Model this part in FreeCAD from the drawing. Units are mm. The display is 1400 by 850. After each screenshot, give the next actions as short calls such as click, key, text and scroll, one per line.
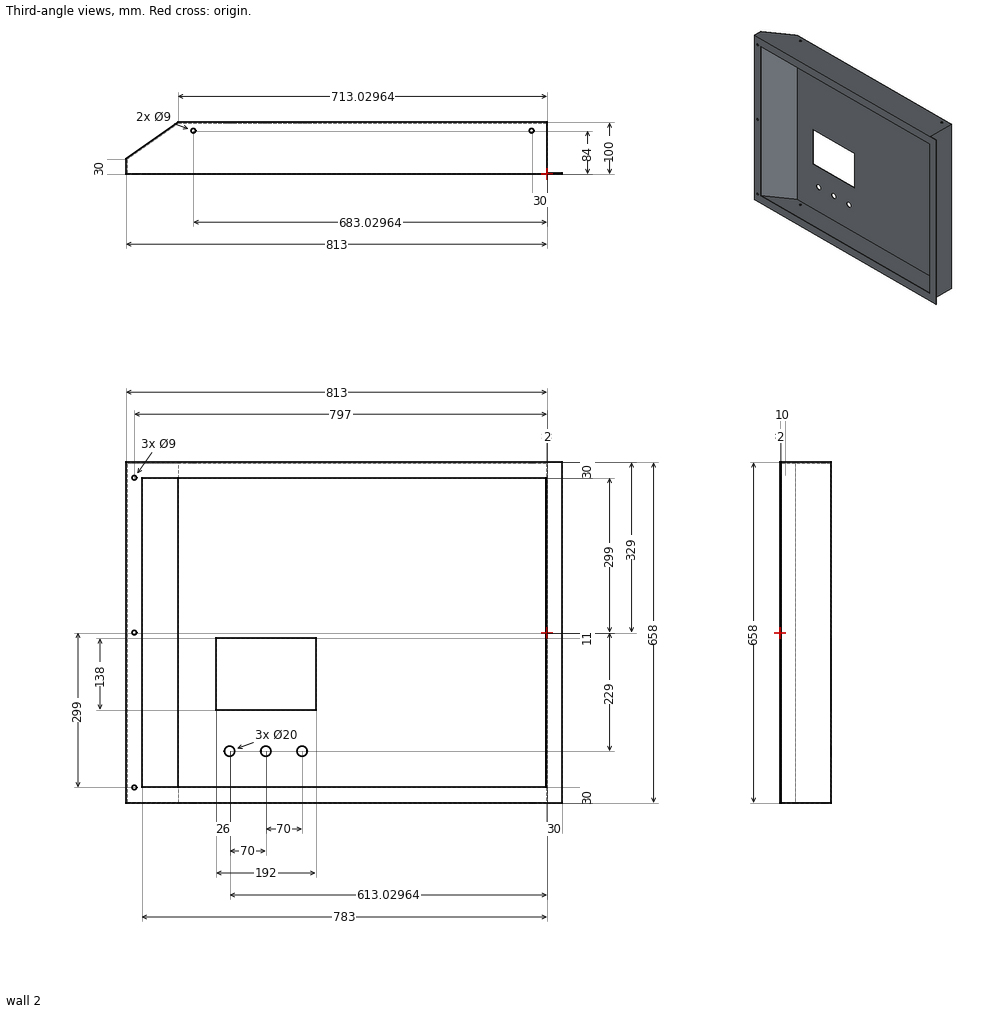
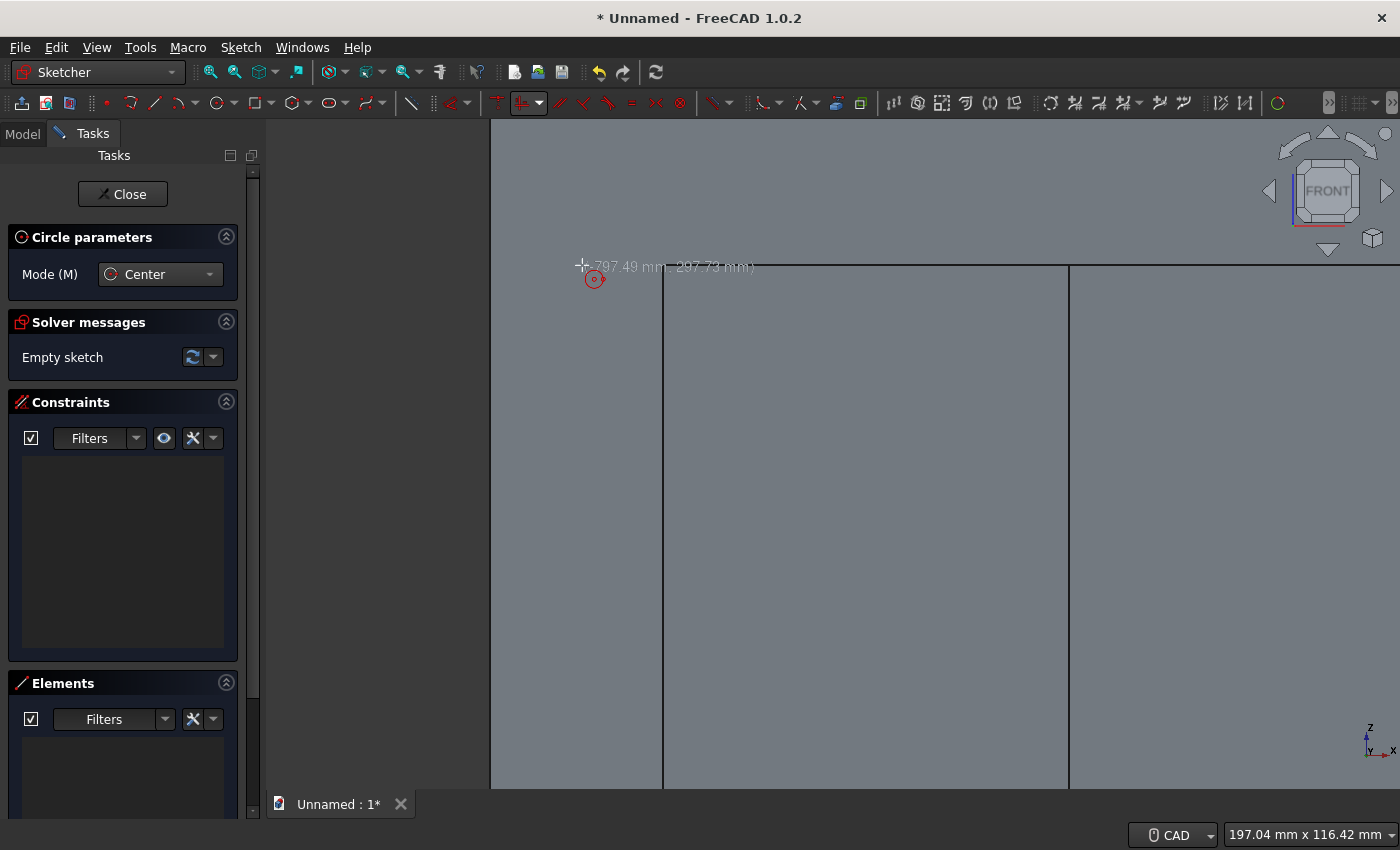
scroll(436, 214, down, 10)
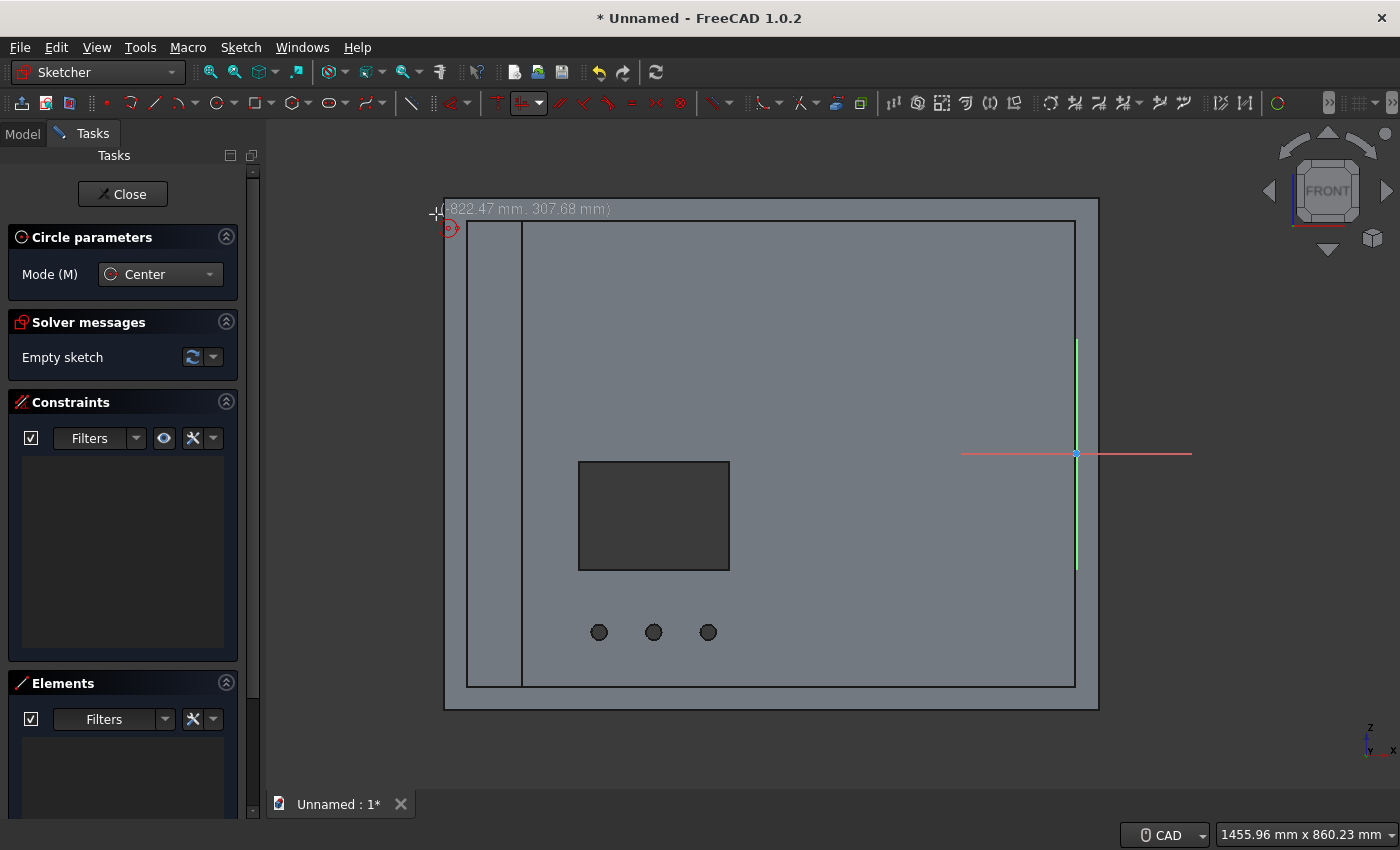
click(456, 221)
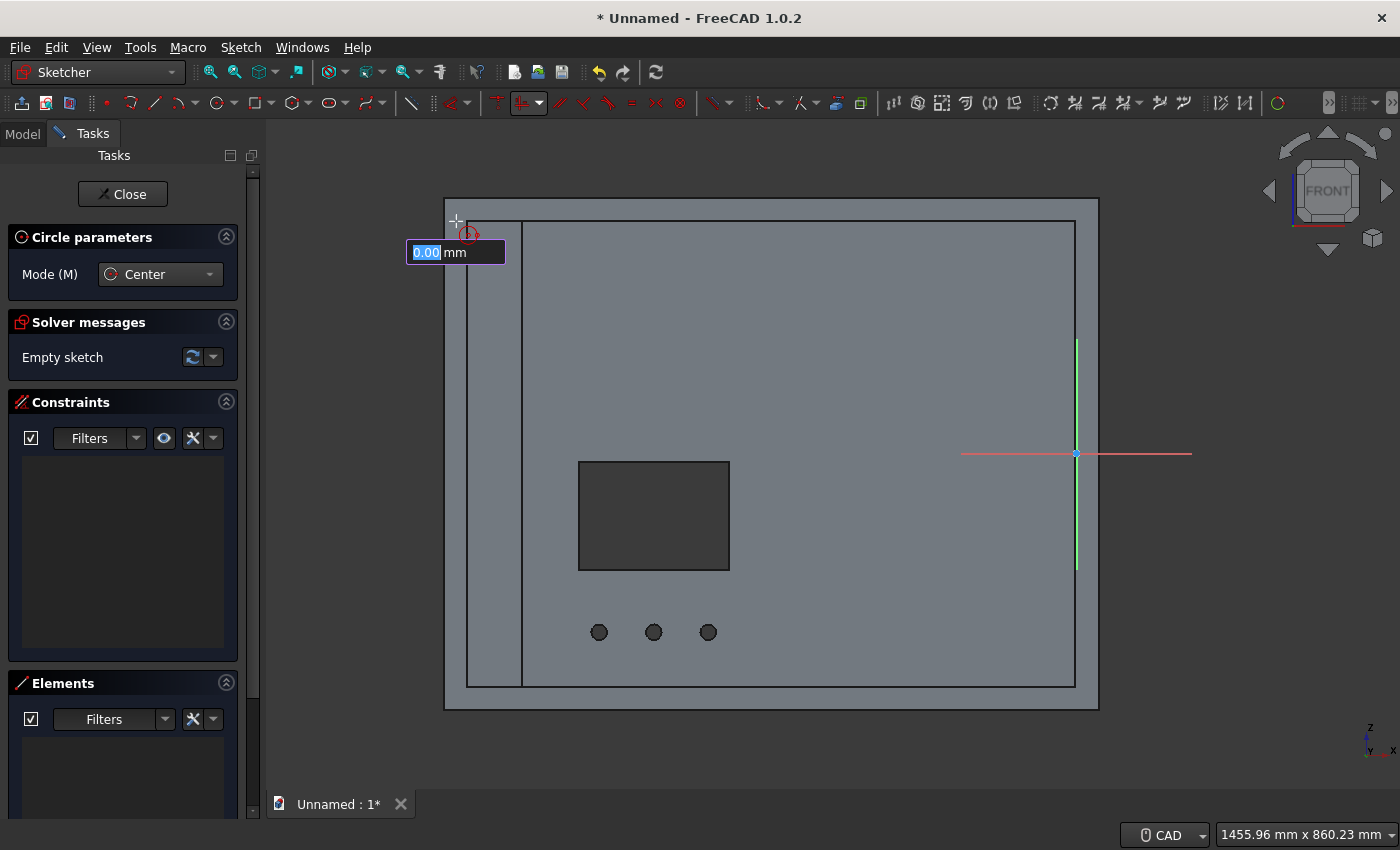
scroll(458, 219, up, 8)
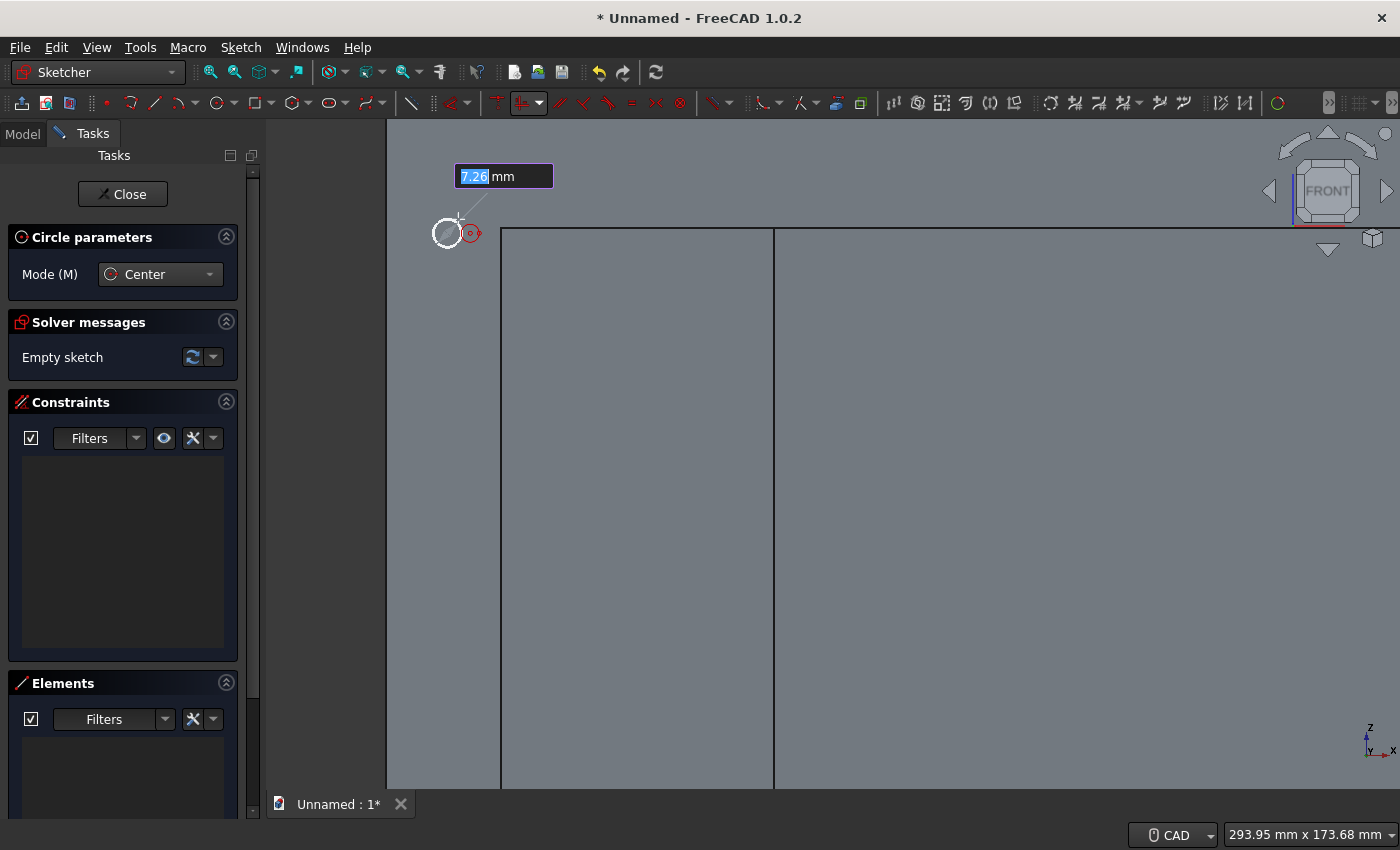
click(460, 216)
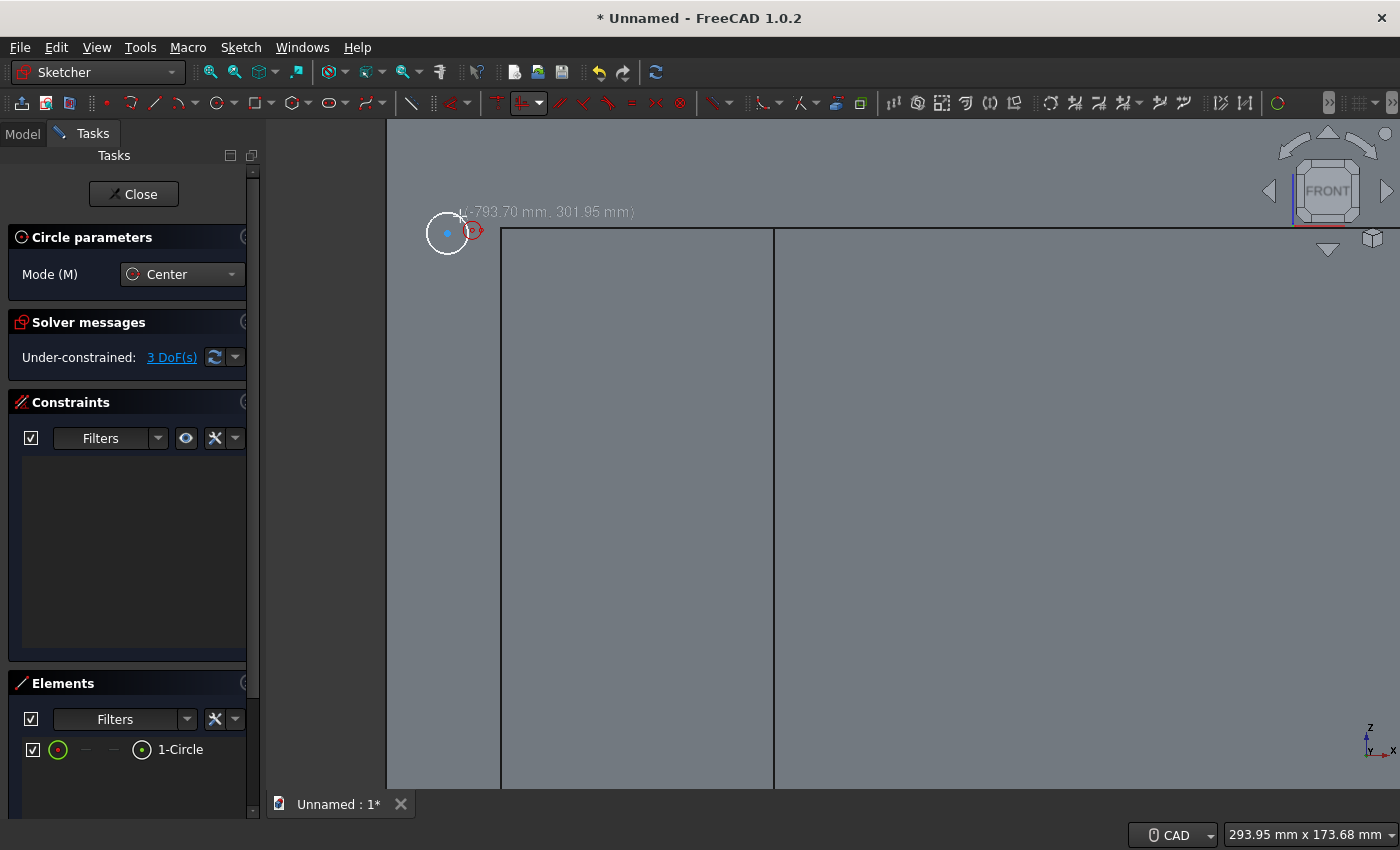
scroll(458, 219, down, 8)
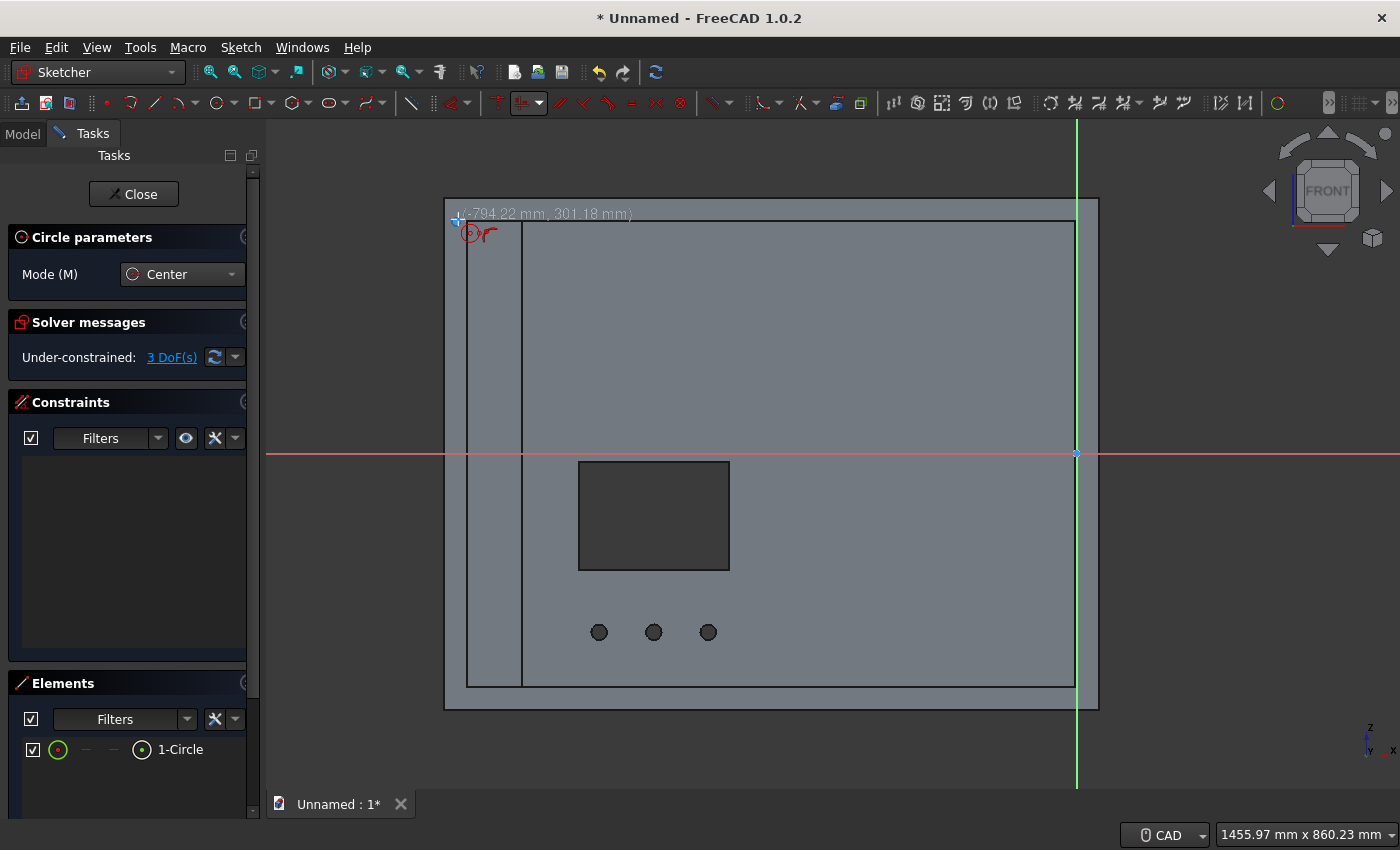
scroll(456, 687, up, 10)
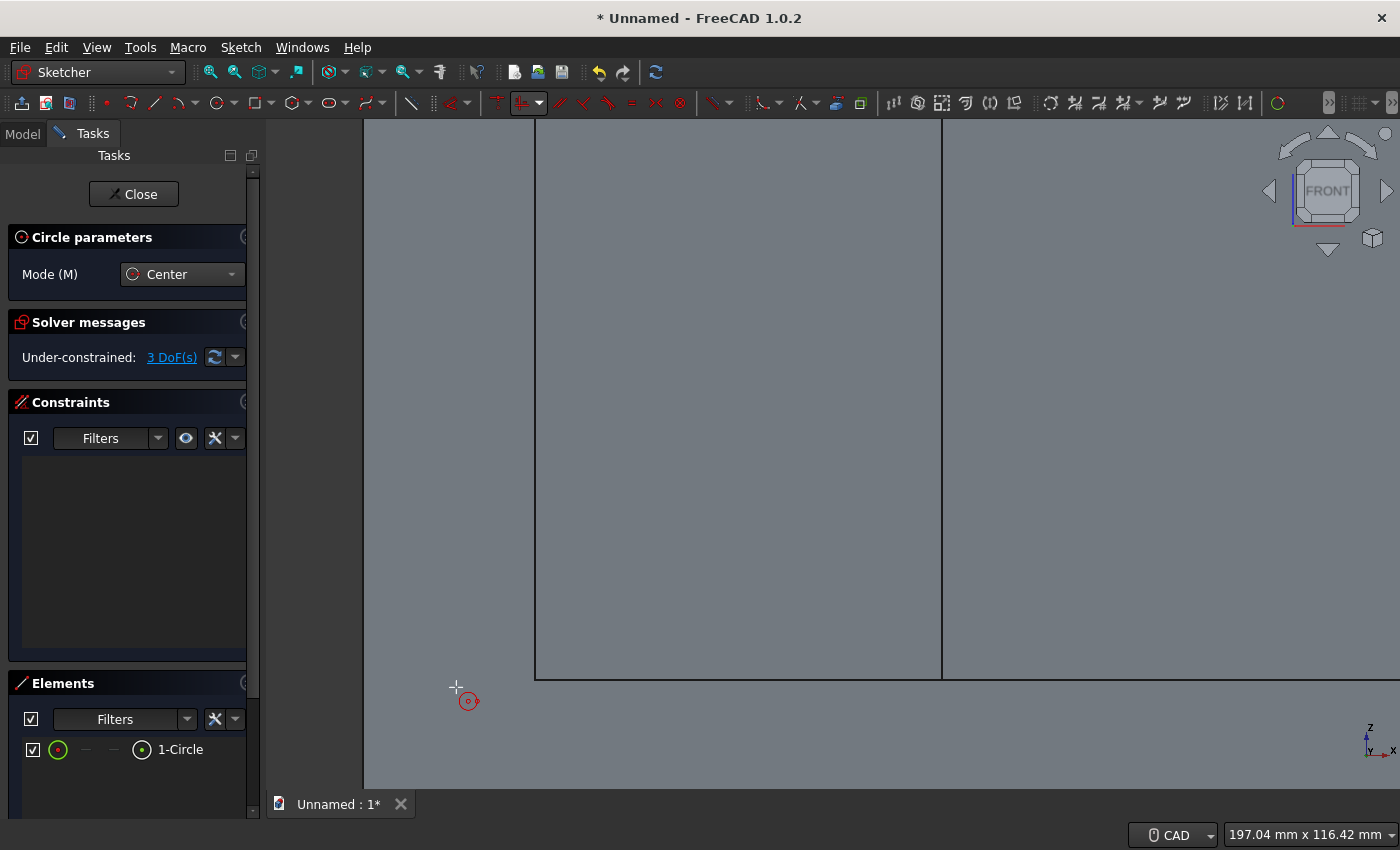
scroll(456, 688, down, 10)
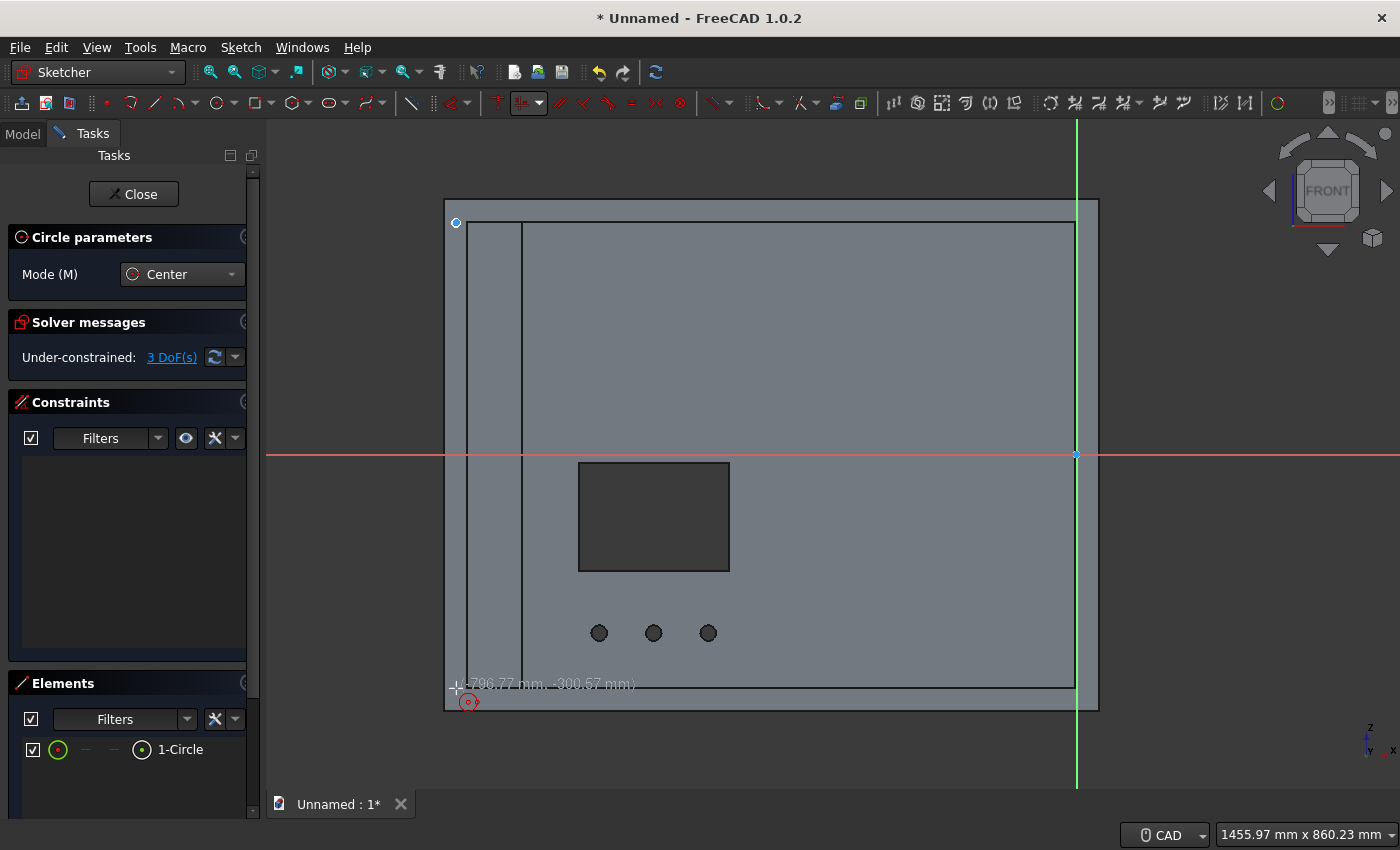
click(456, 688)